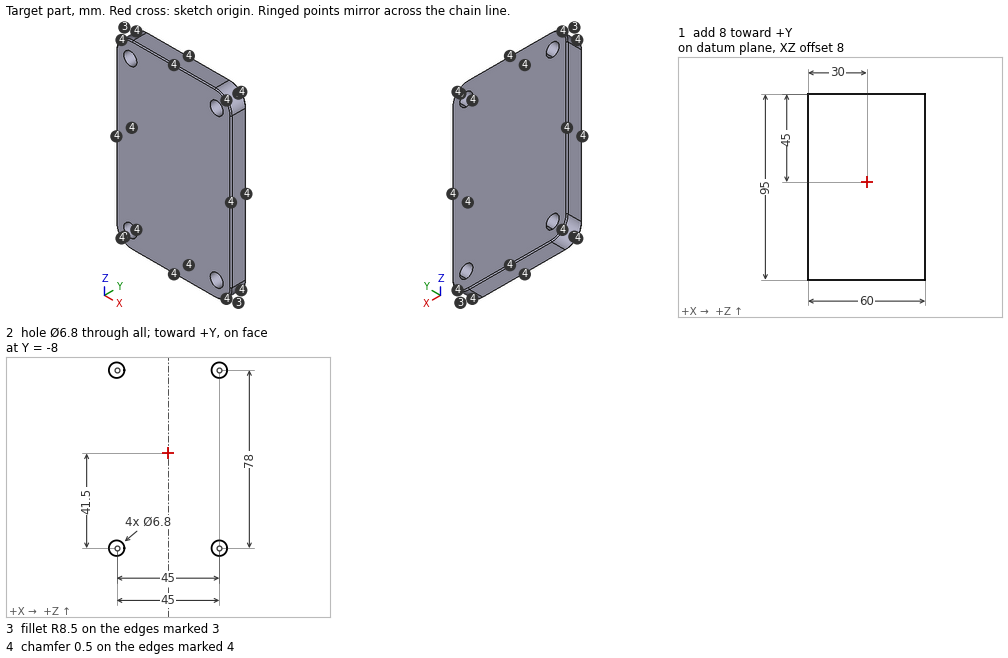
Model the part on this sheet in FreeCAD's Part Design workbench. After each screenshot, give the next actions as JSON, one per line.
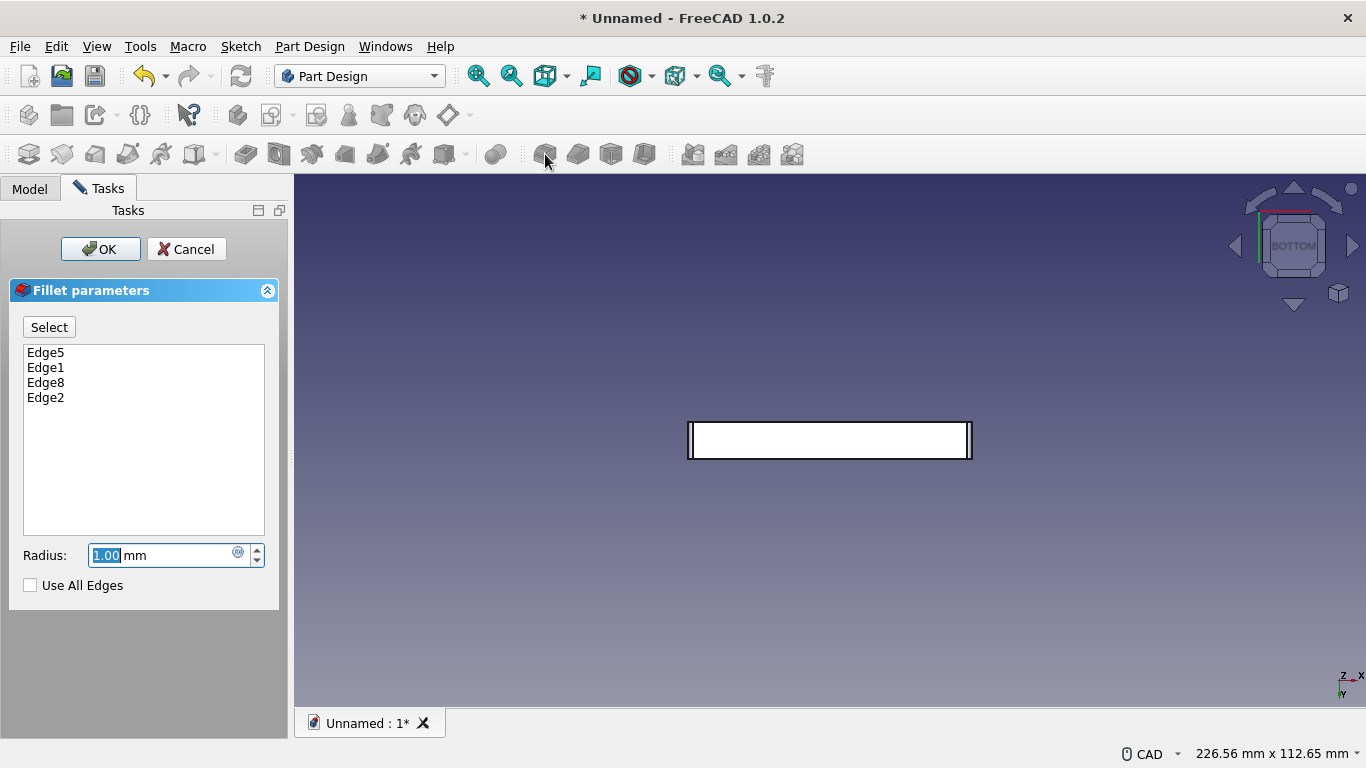
{"action": "type", "text": "8.5"}
{"action": "key", "text": "Tab"}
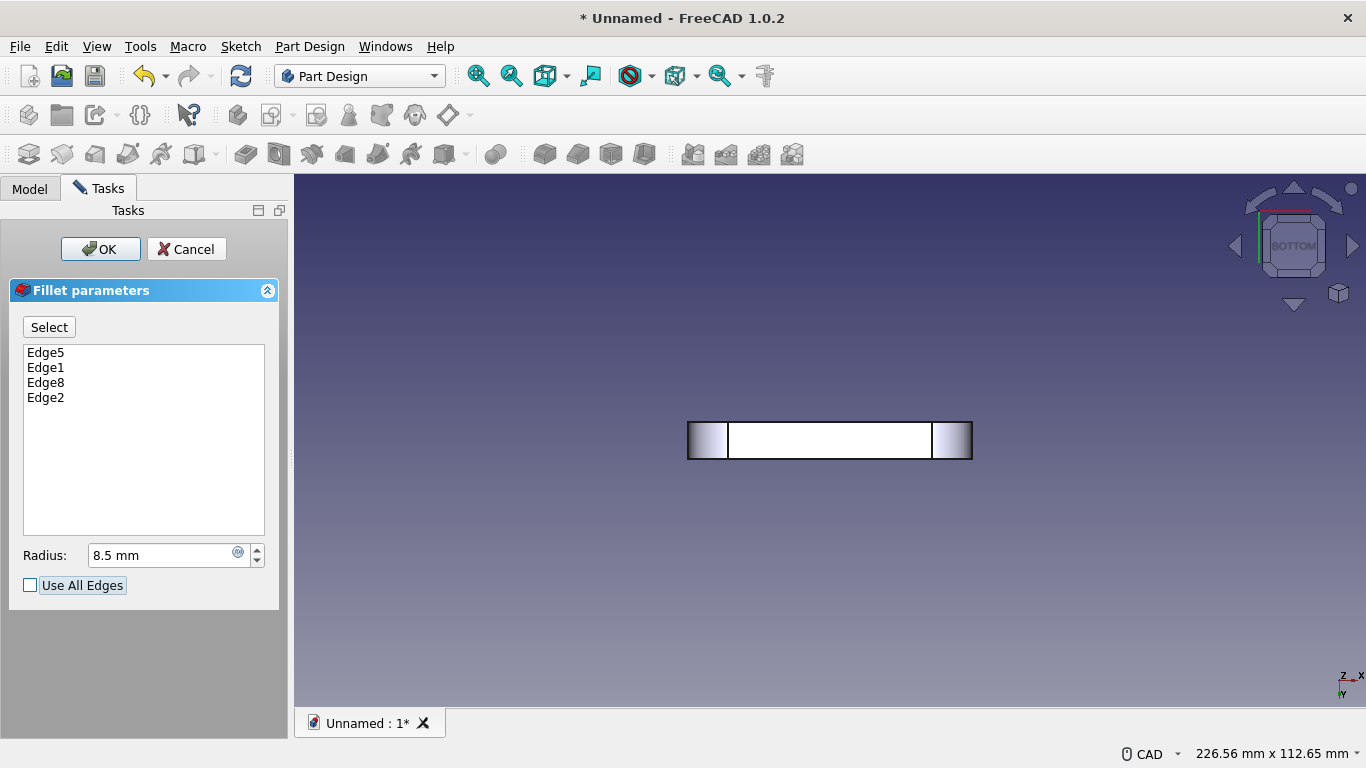
{"action": "left_click", "coordinate": [101, 249]}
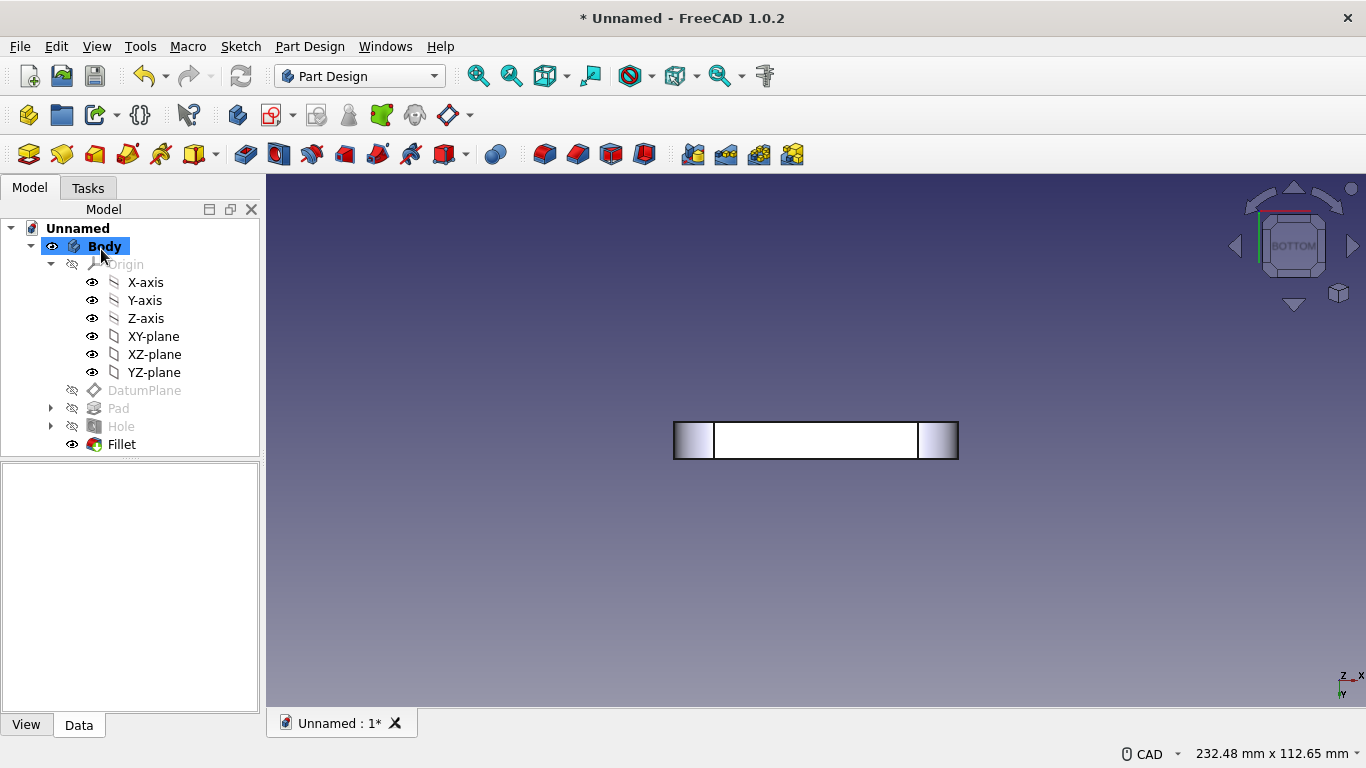
{"action": "key", "text": "v f"}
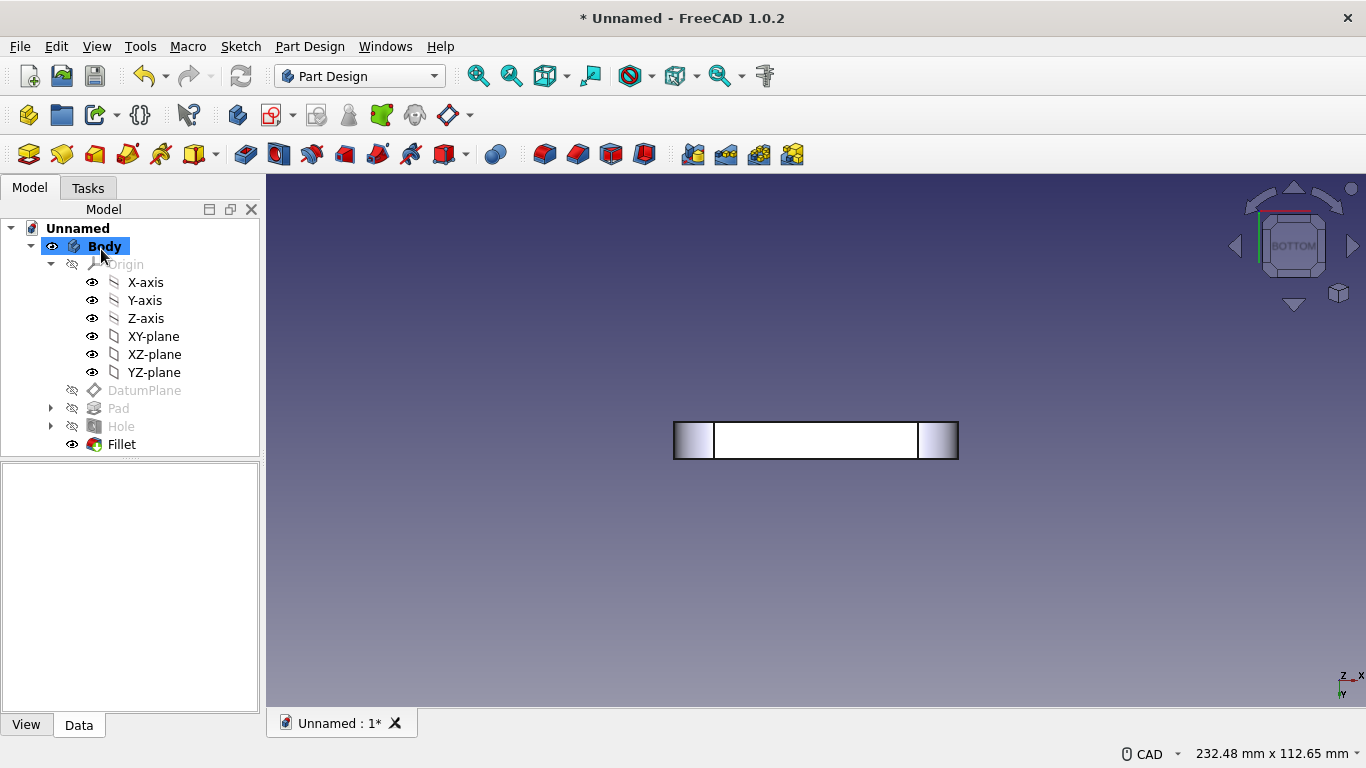
{"action": "left_click", "coordinate": [816, 421]}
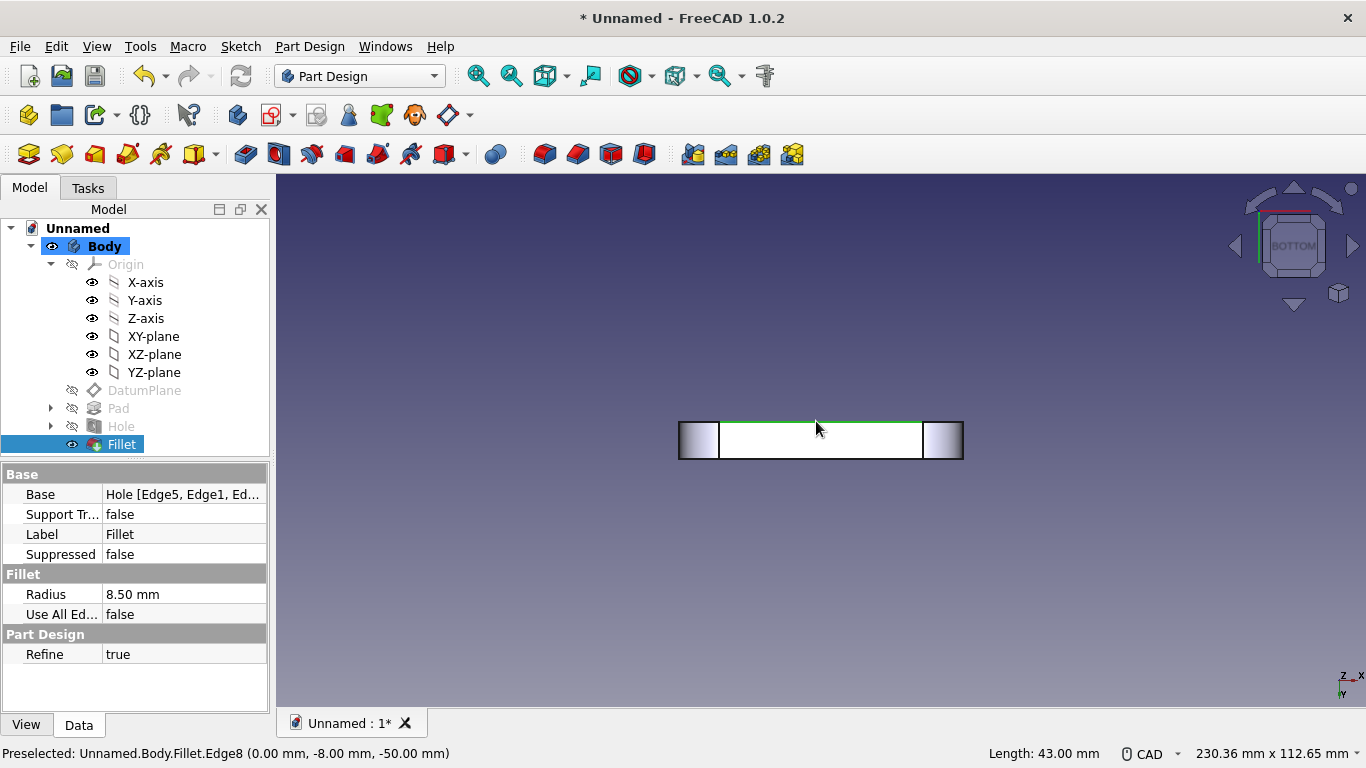
{"action": "left_click", "coordinate": [691, 421], "text": "ctrl"}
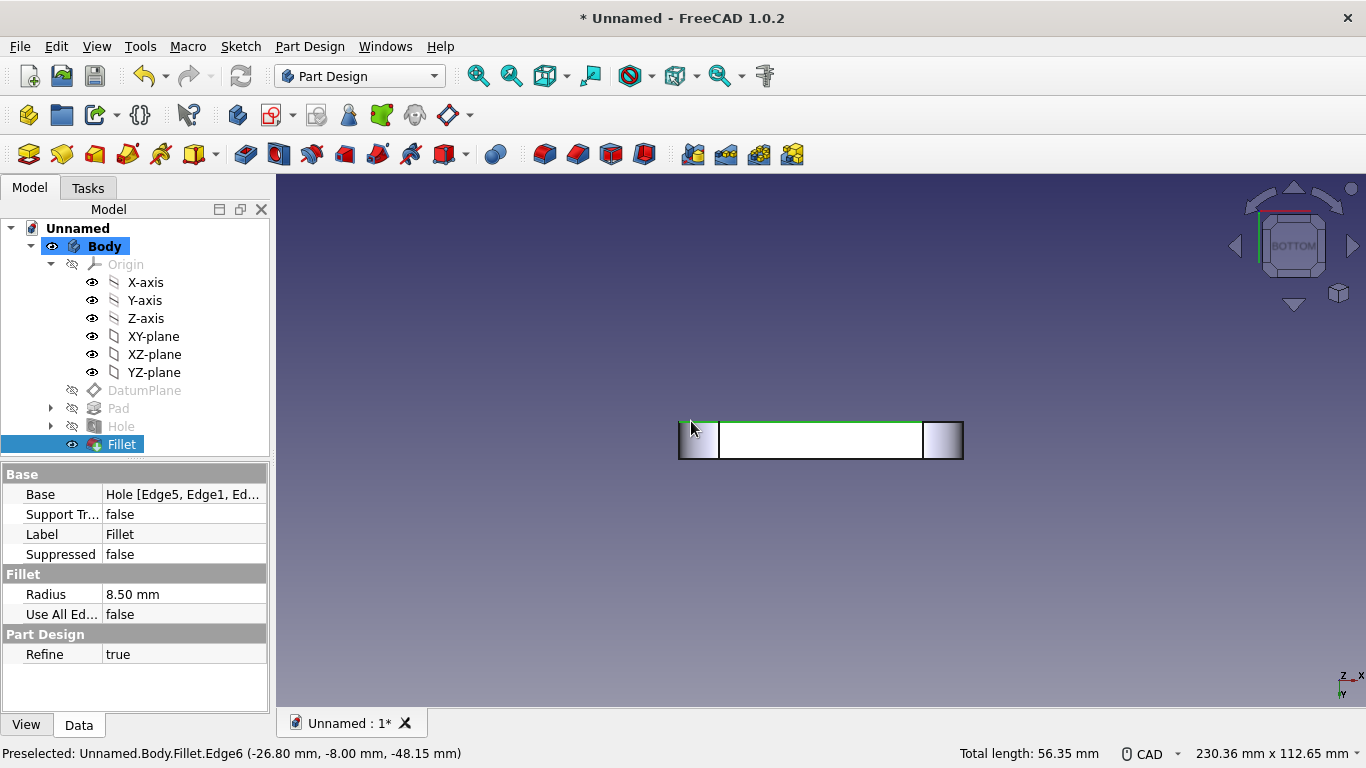
{"action": "left_click", "coordinate": [951, 421], "text": "ctrl"}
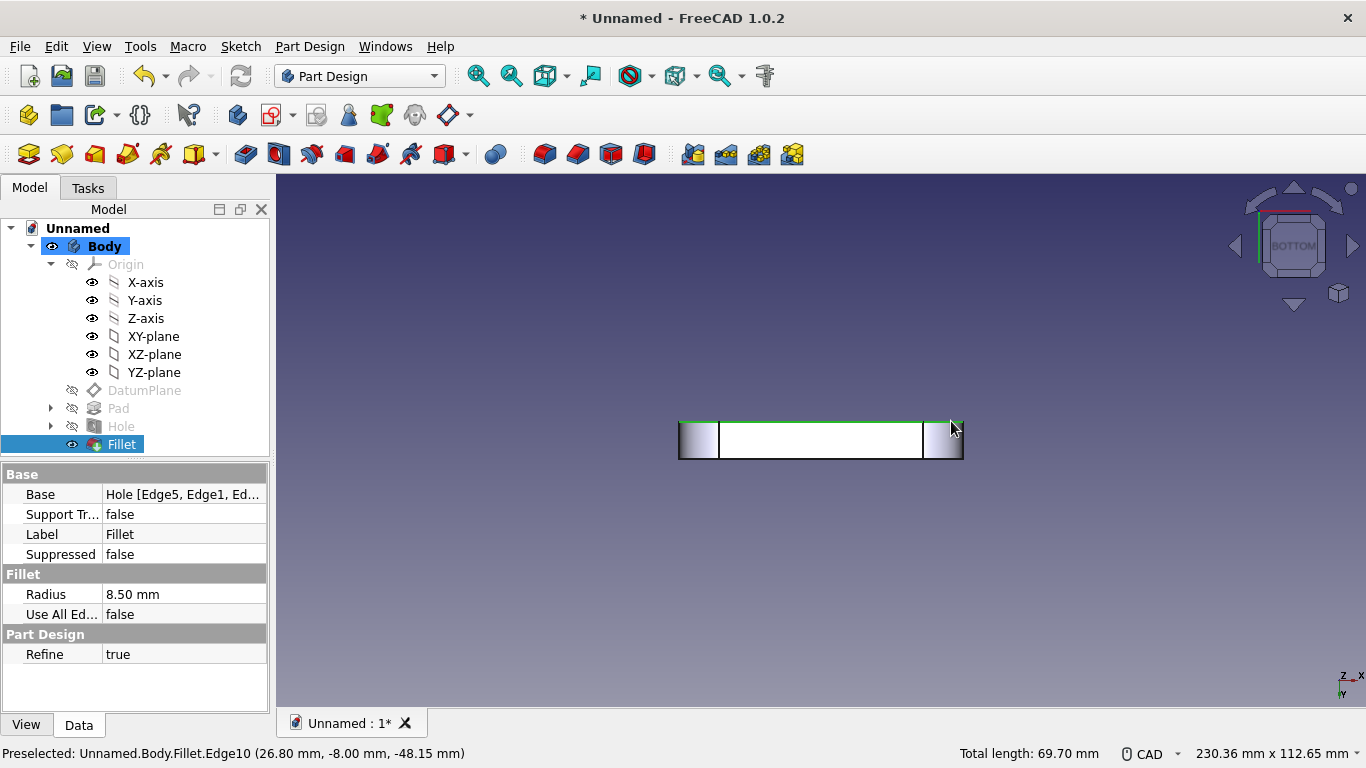
{"action": "left_click", "coordinate": [681, 458], "text": "ctrl"}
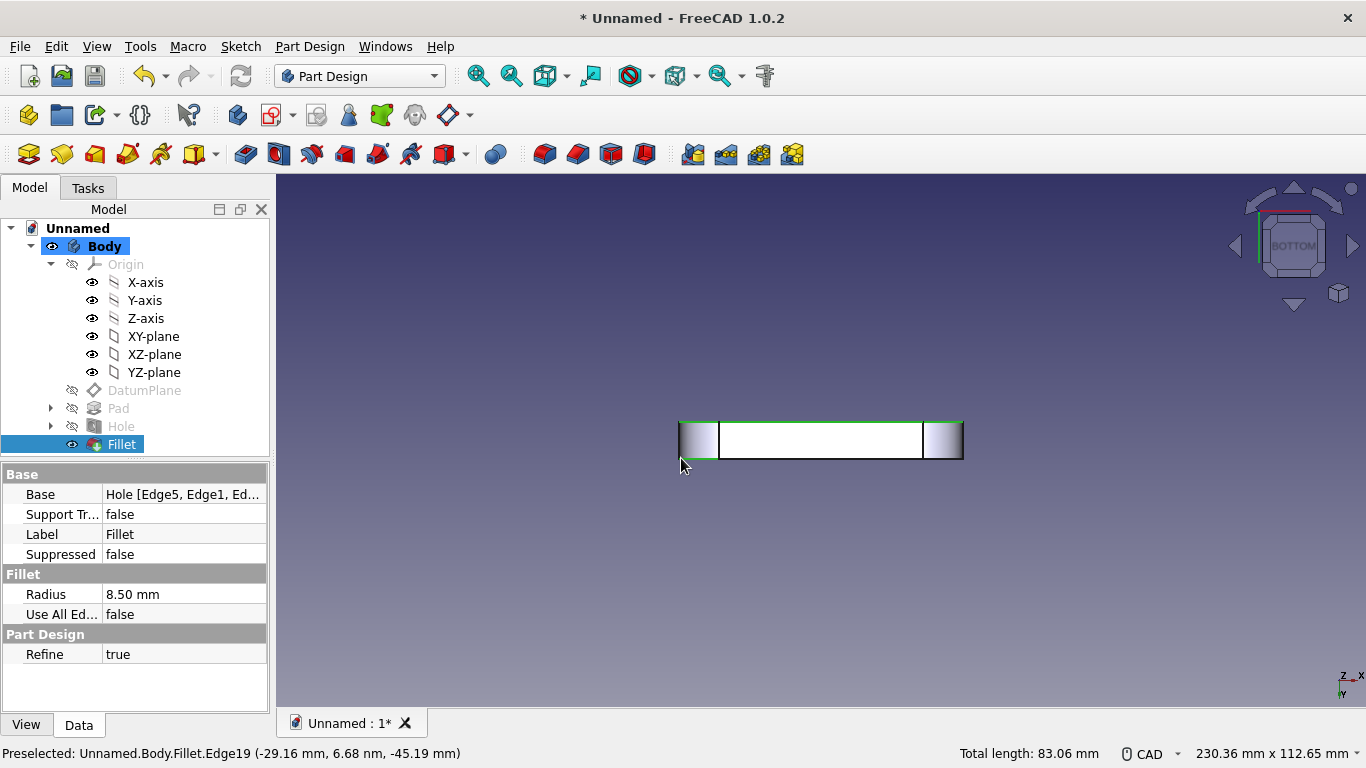
{"action": "left_click", "coordinate": [935, 458], "text": "ctrl"}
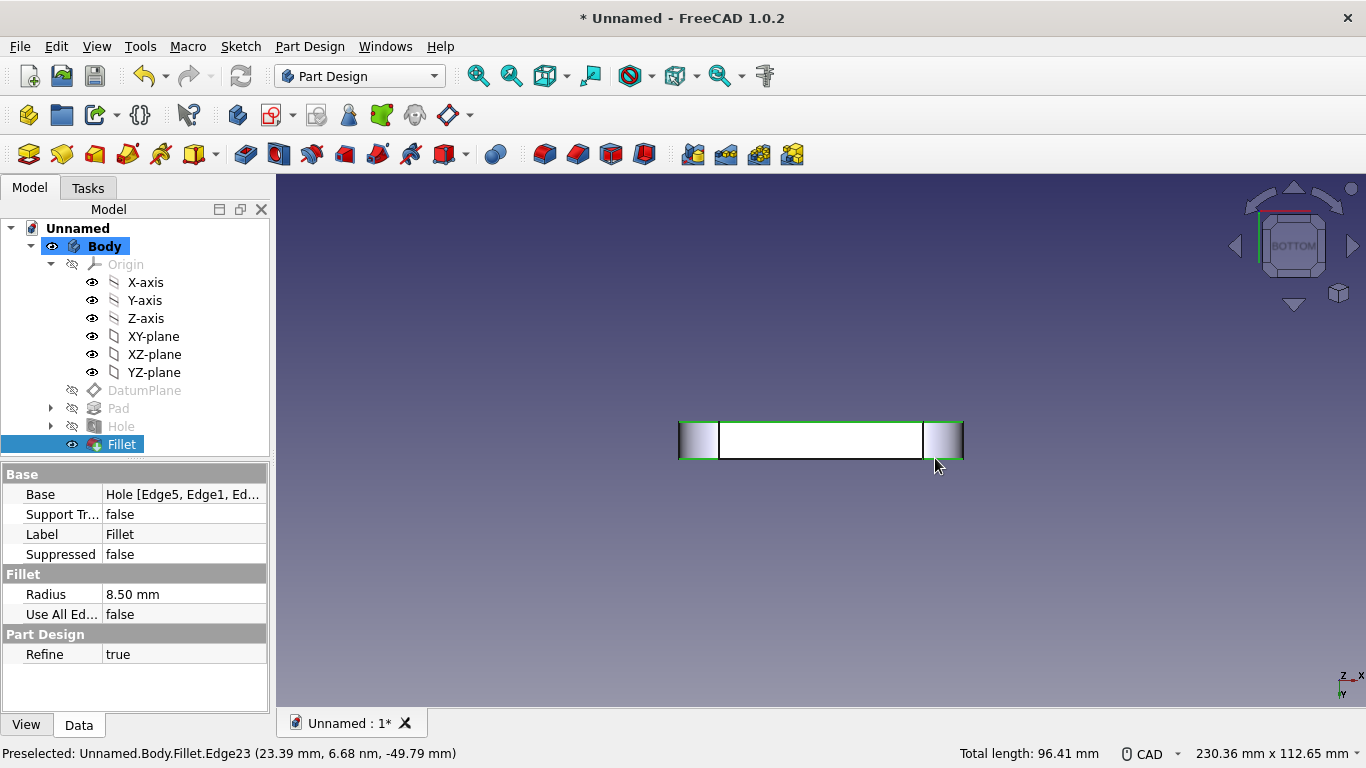
{"action": "key", "text": "0"}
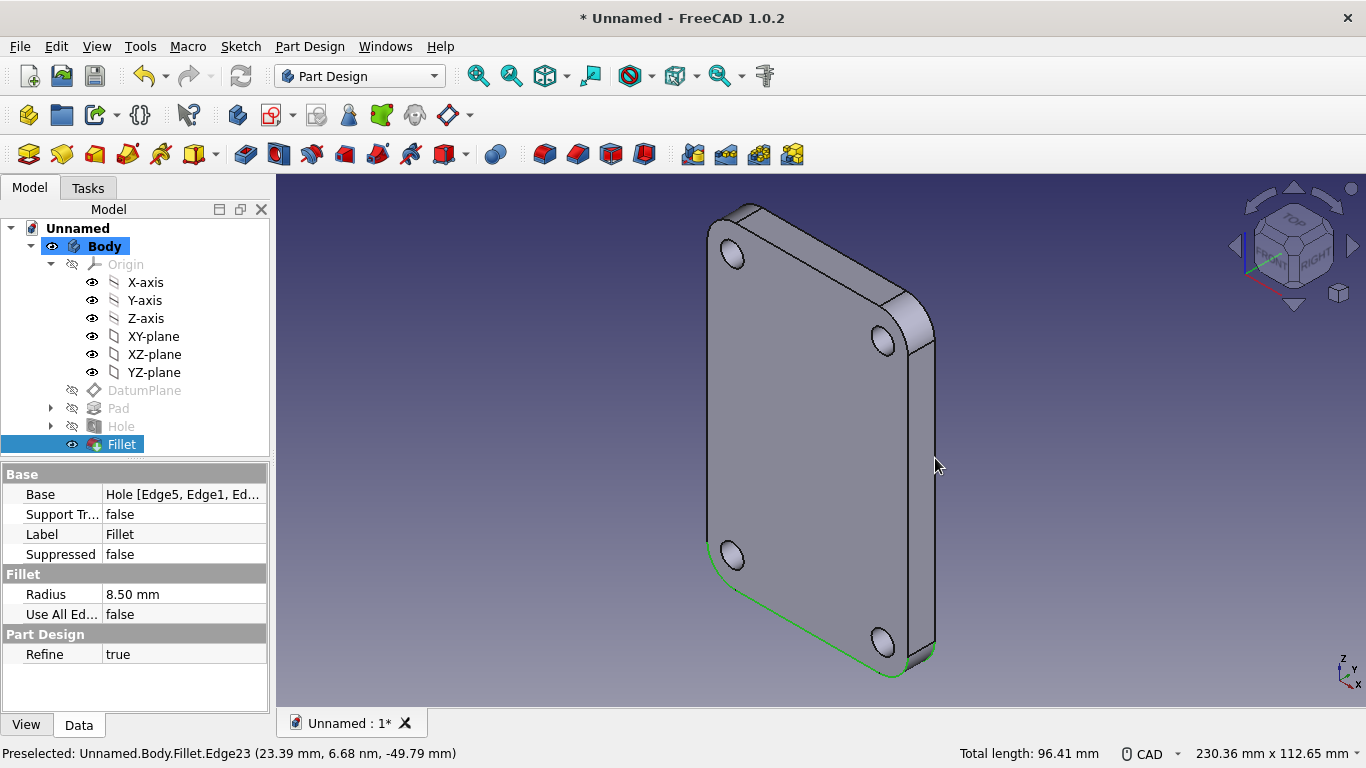
{"action": "left_click", "coordinate": [908, 505], "text": "ctrl"}